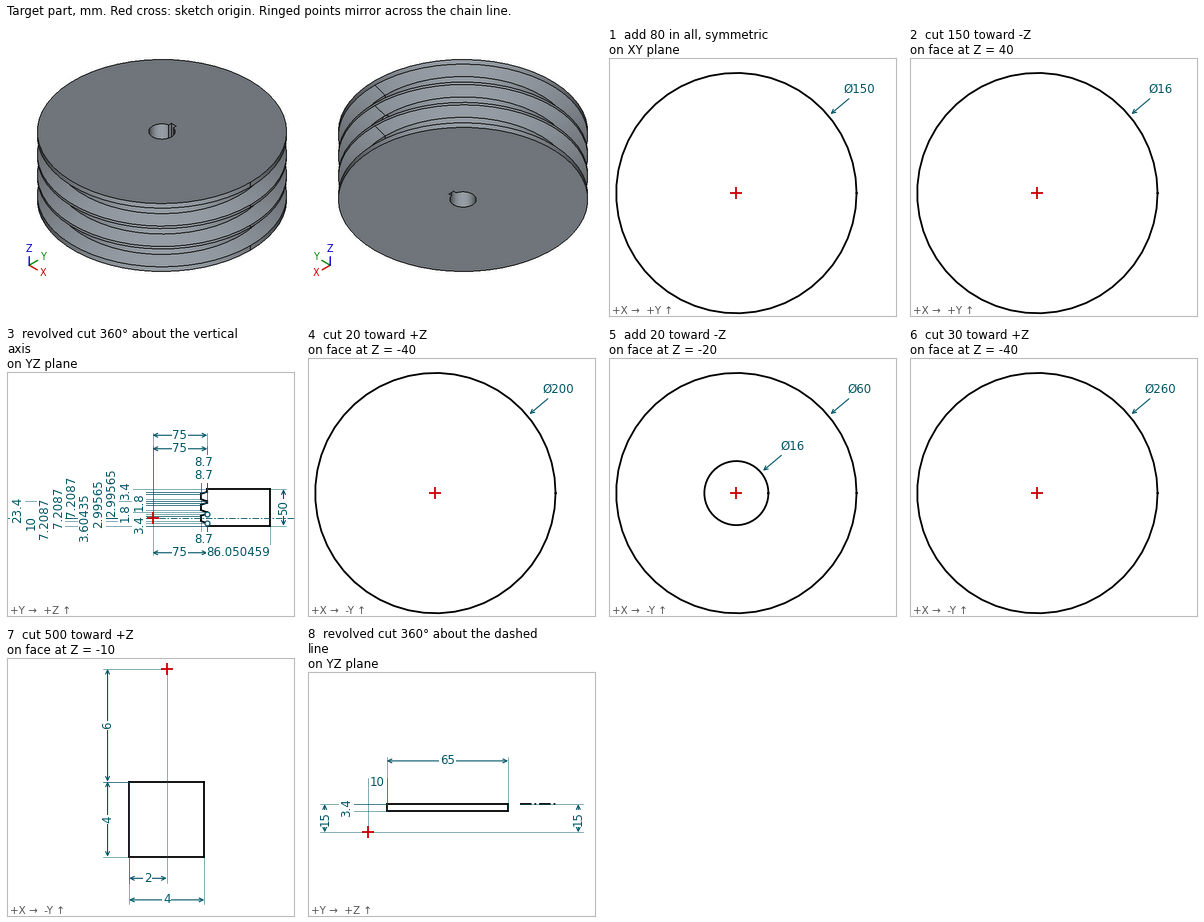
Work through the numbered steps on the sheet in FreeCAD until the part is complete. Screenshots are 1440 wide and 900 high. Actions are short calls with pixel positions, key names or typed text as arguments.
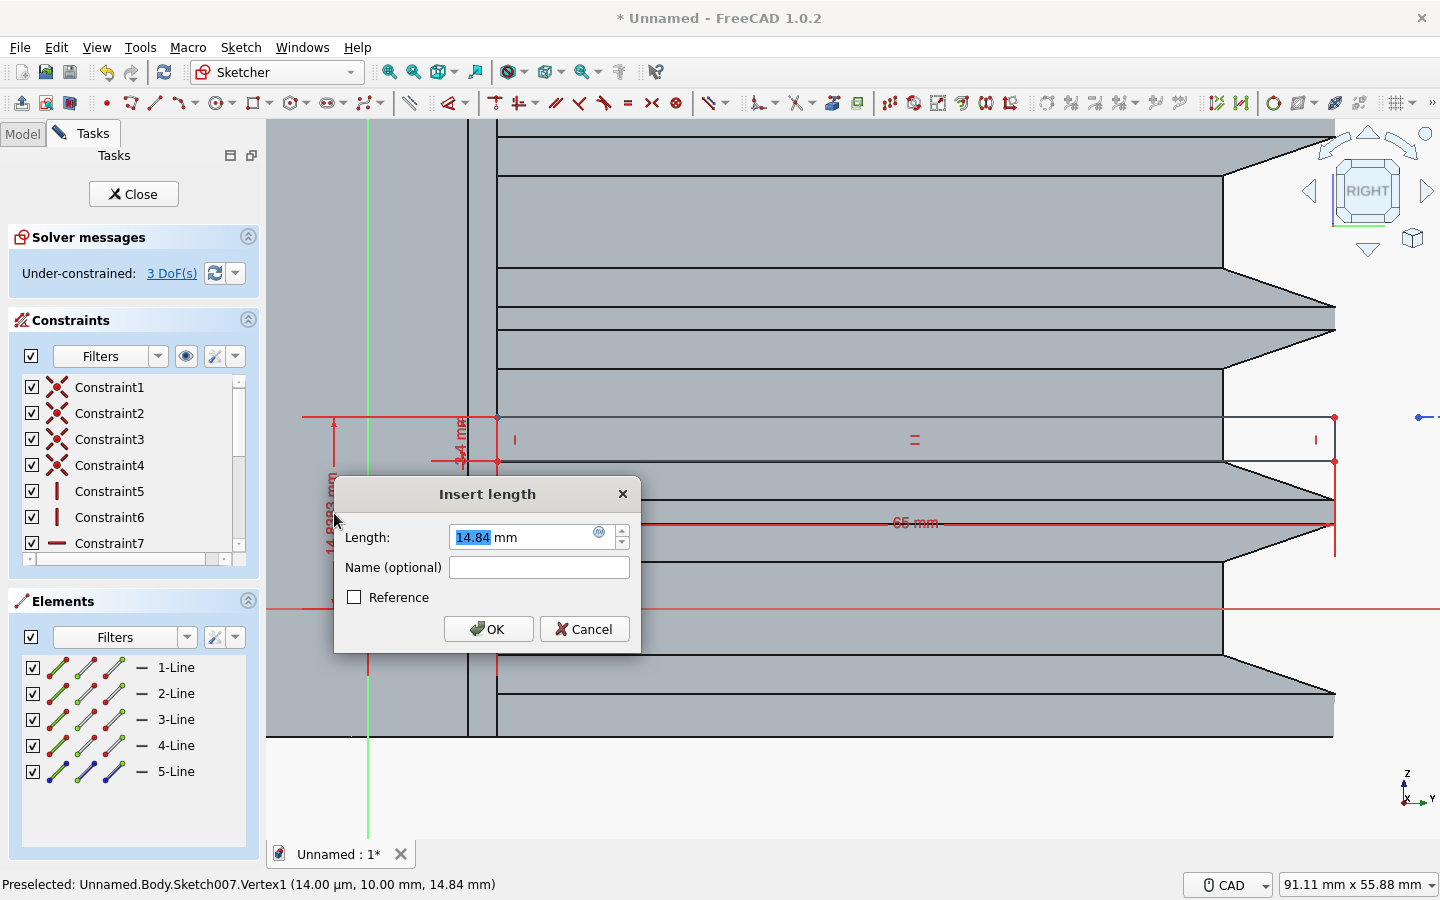
text(15)
key(Return)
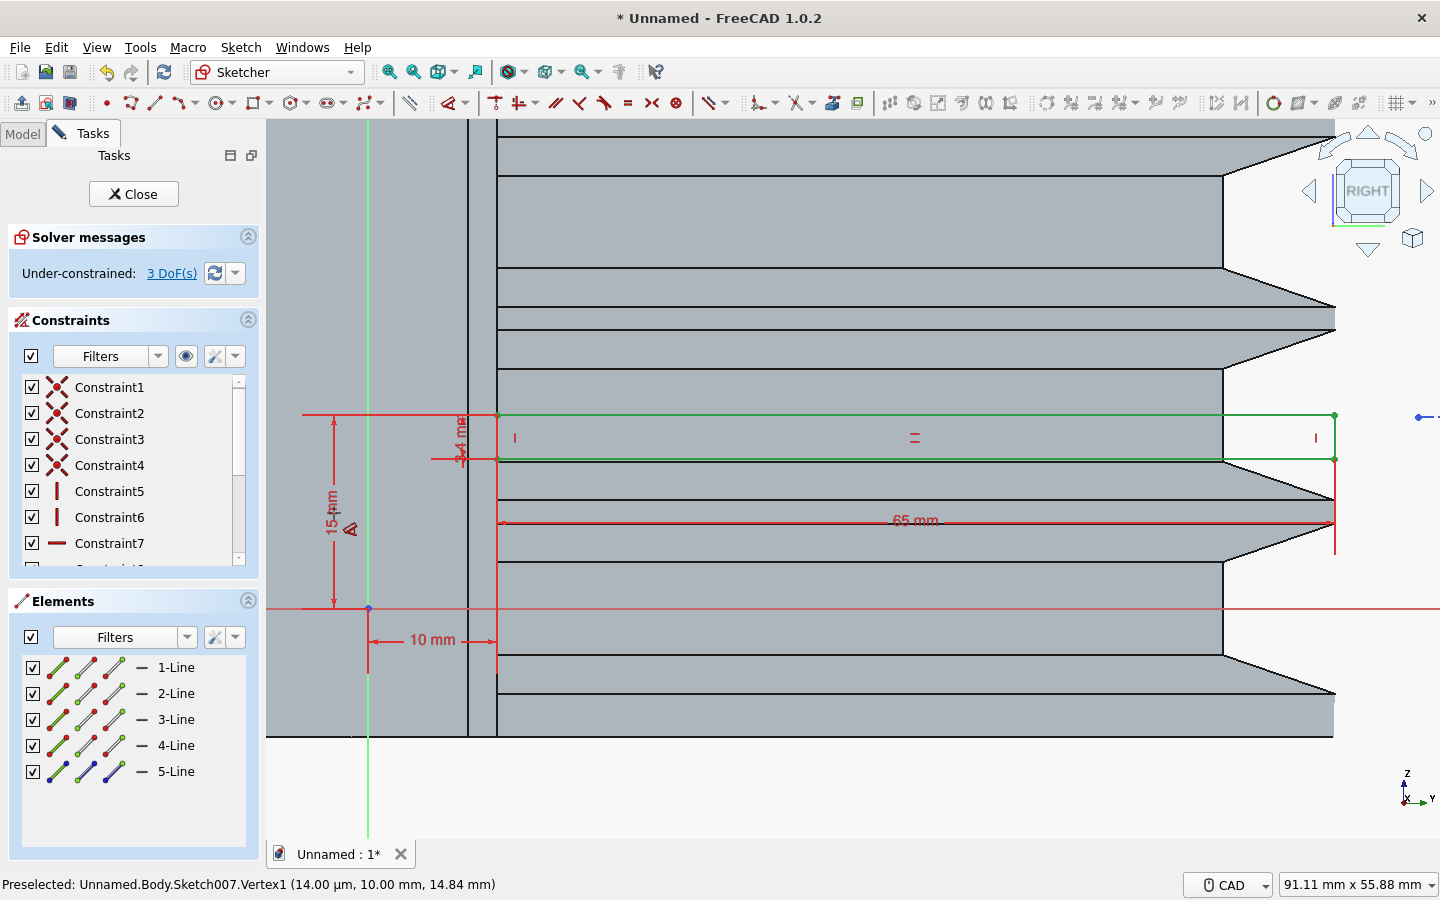
scroll(499, 439, down, 3)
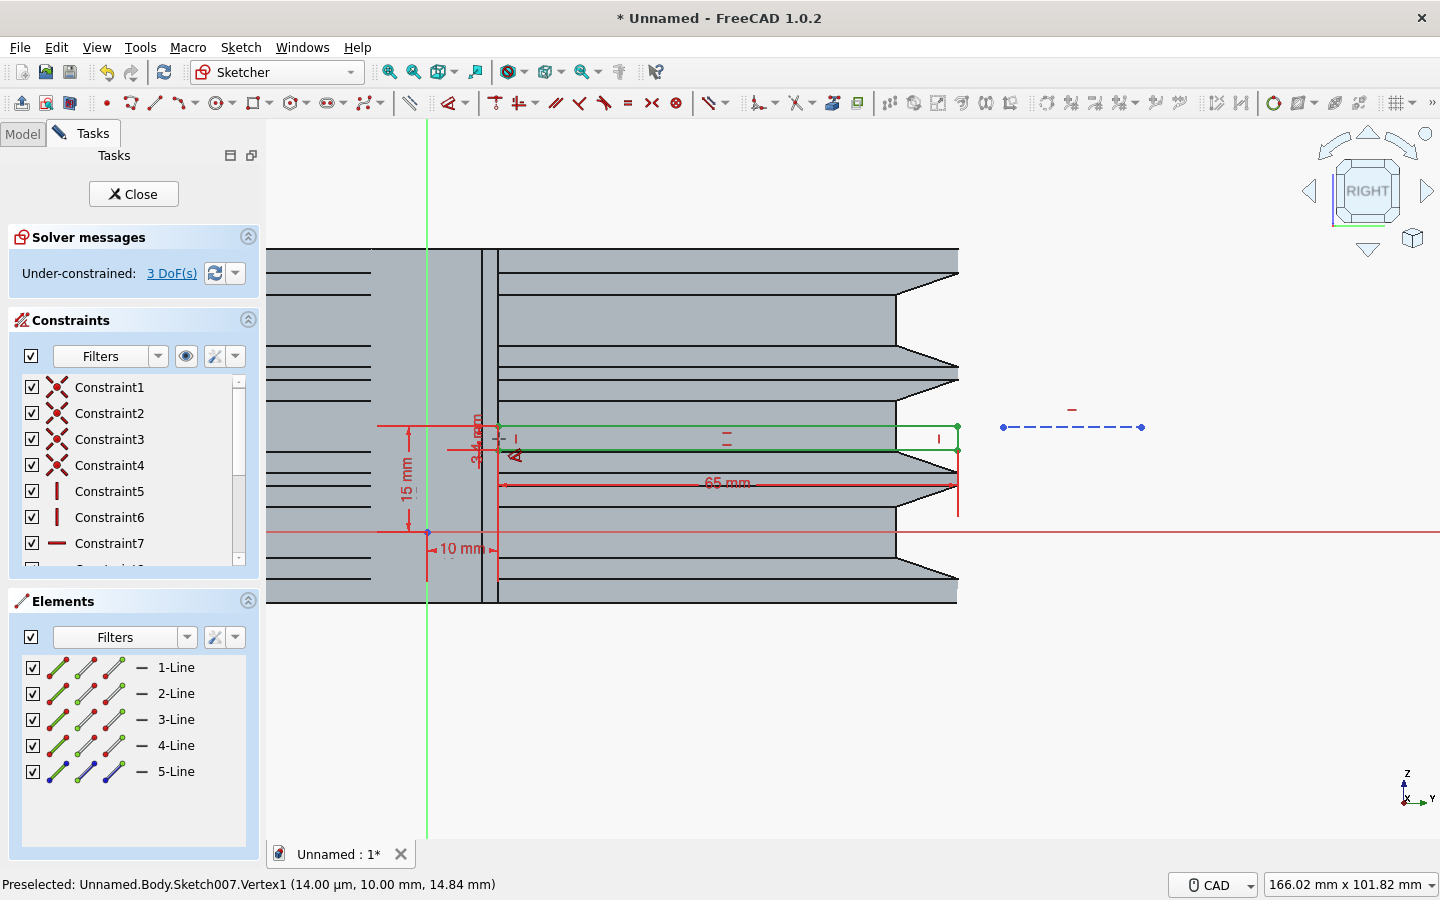
click(1004, 427)
click(393, 456)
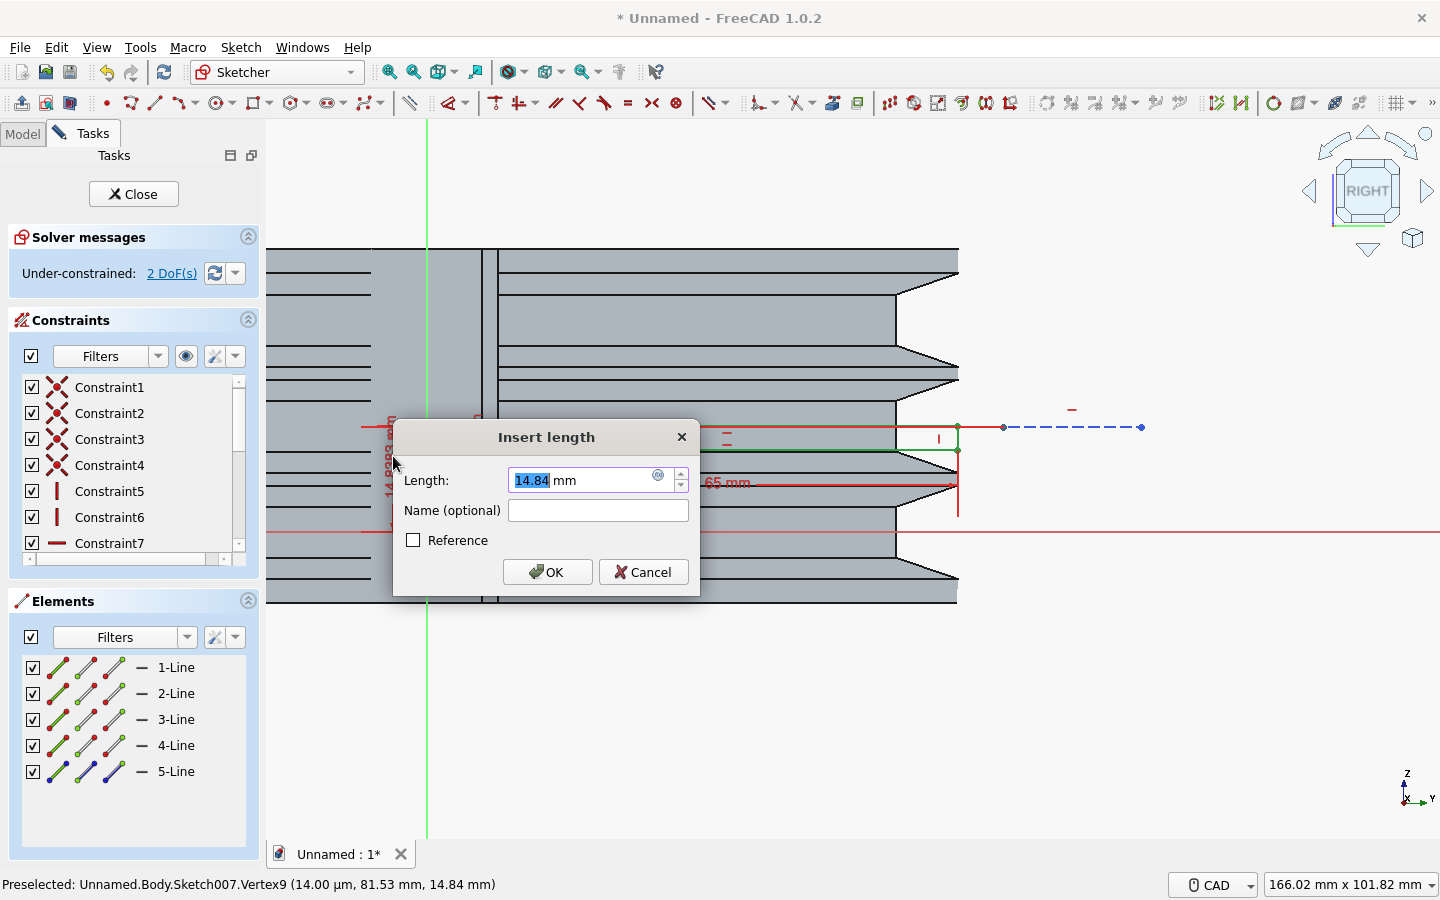
text(15)
key(Return)
key(Escape)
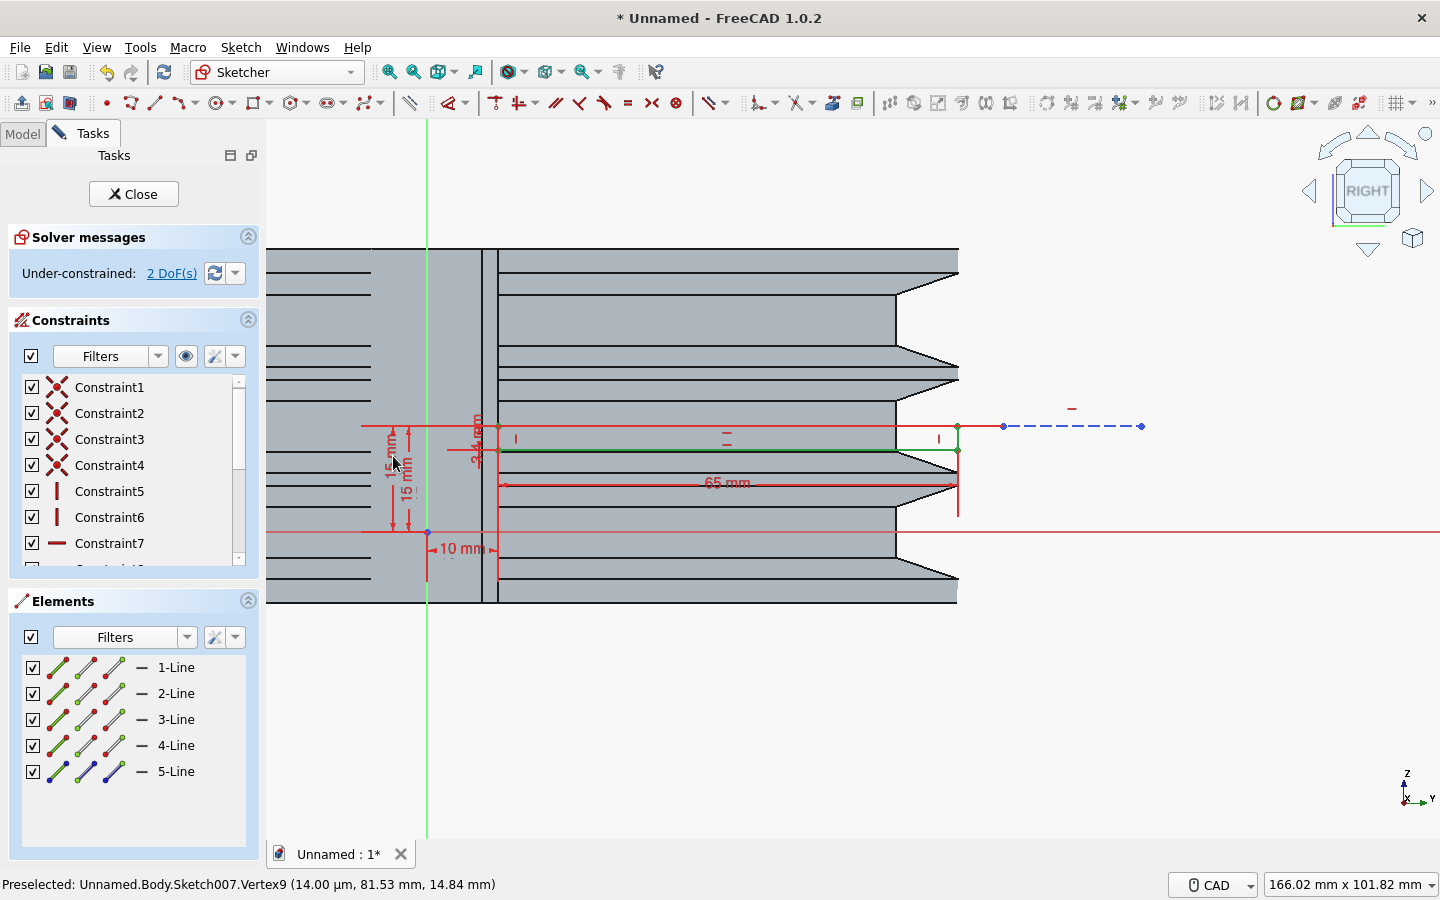
click(134, 194)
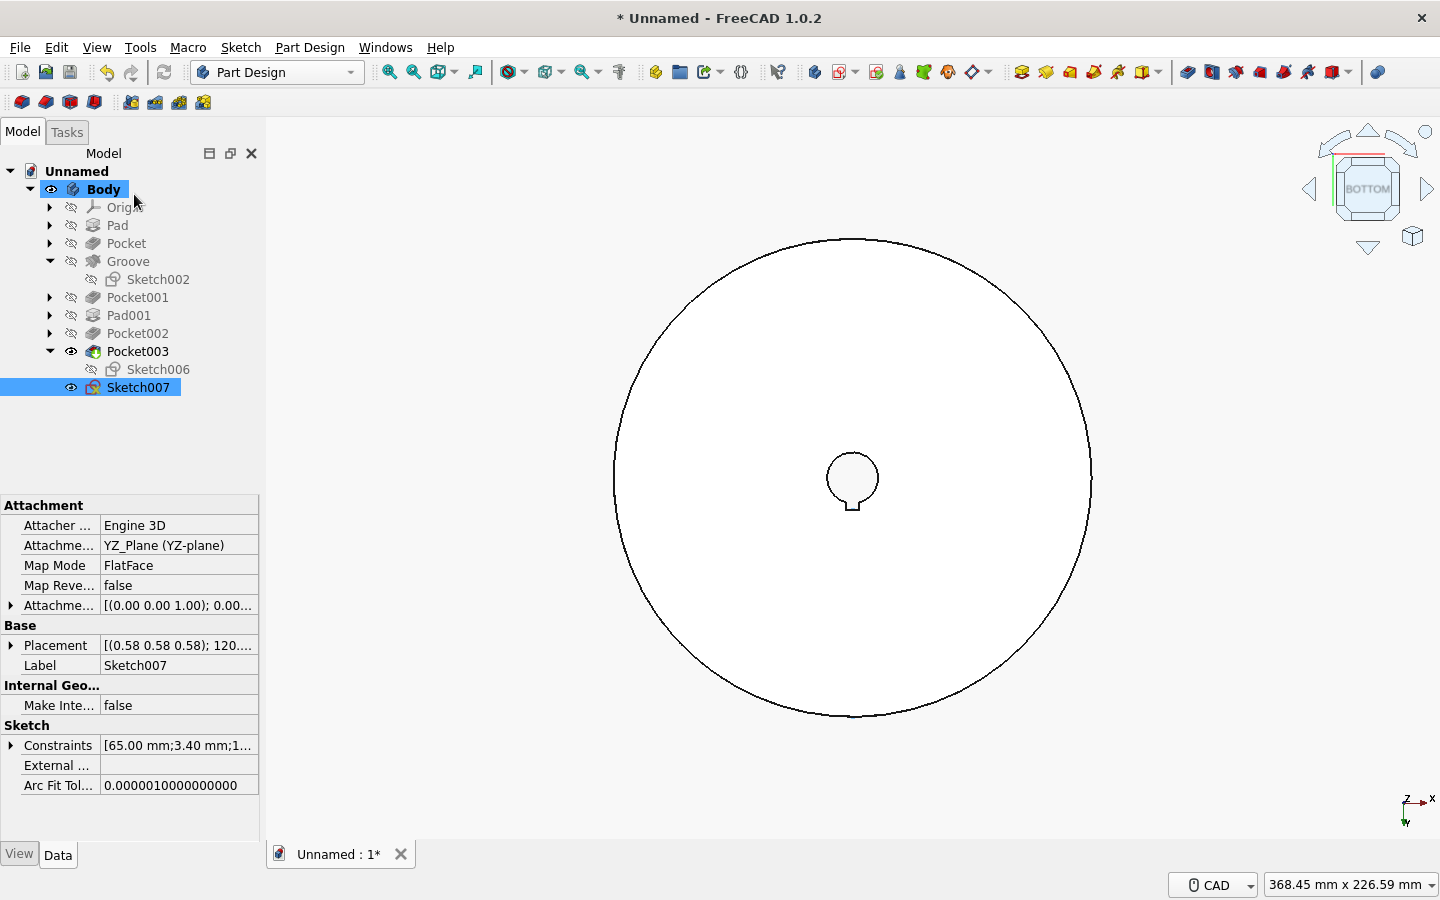
click(1236, 72)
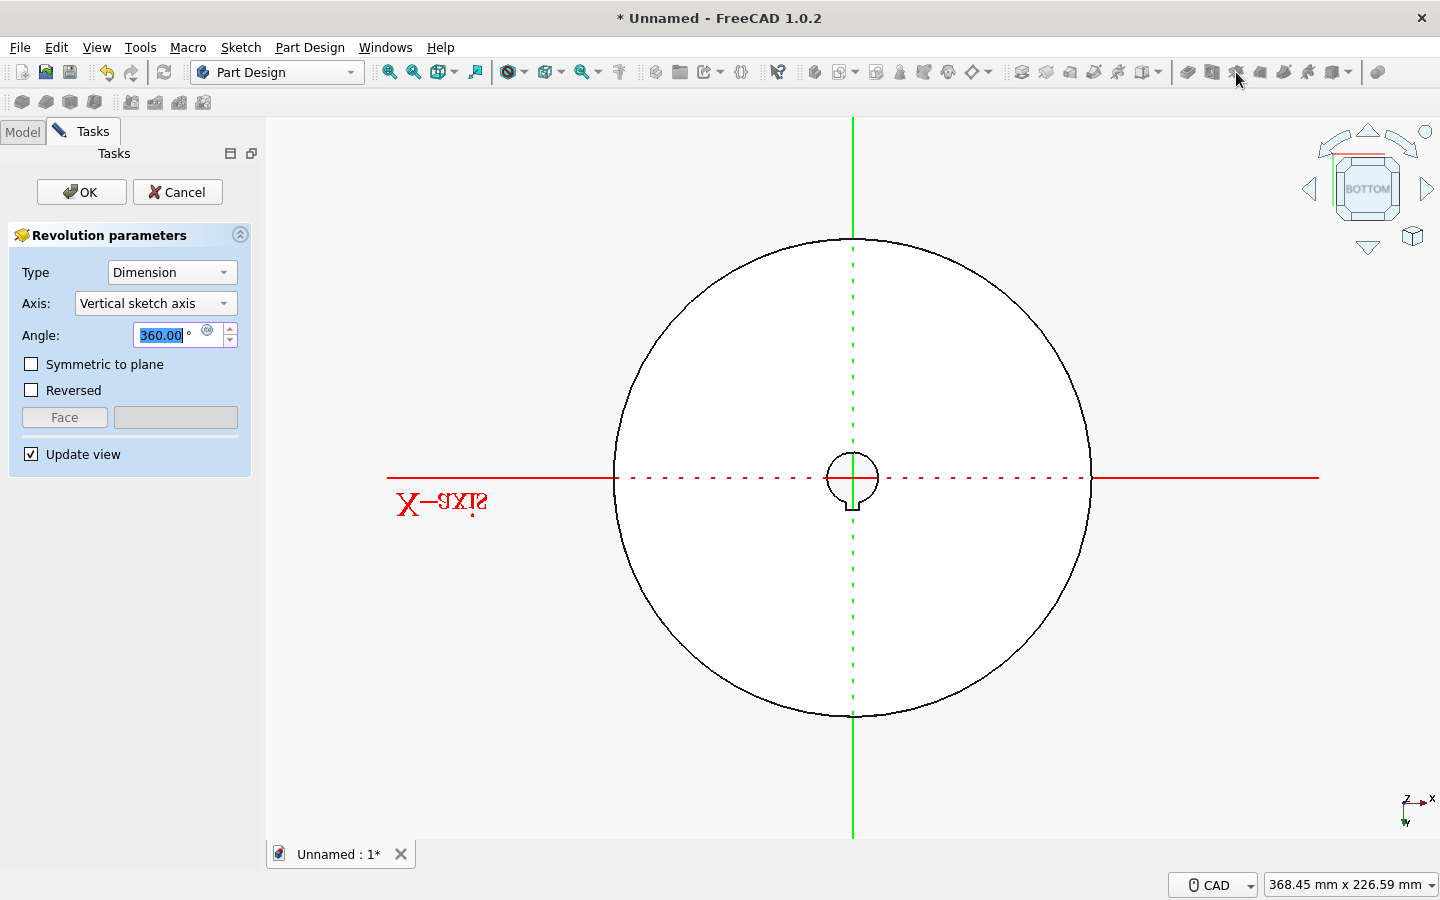
click(156, 304)